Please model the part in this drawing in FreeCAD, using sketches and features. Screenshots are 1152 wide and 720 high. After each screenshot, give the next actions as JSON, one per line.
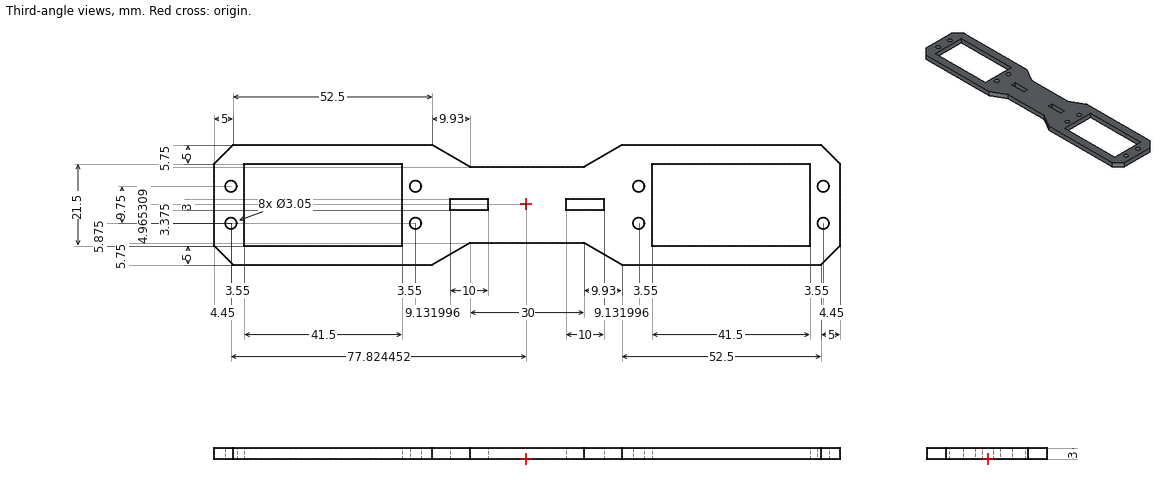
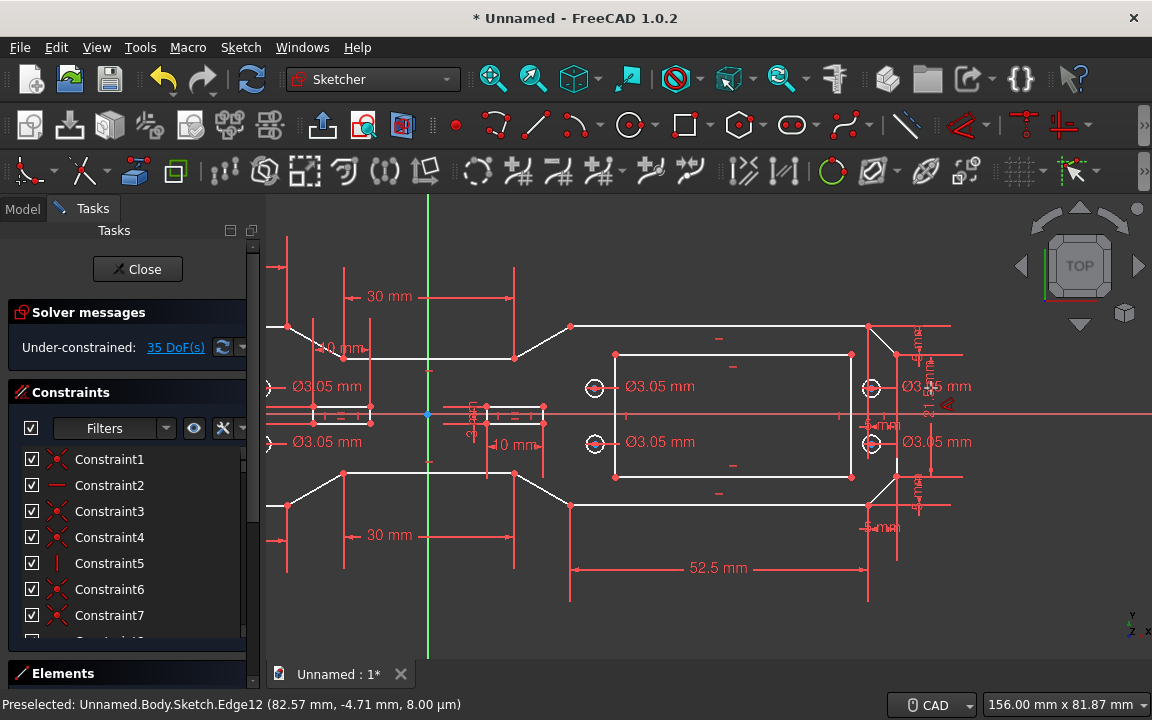
{"action": "left_click", "coordinate": [779, 326]}
{"action": "left_click", "coordinate": [719, 292]}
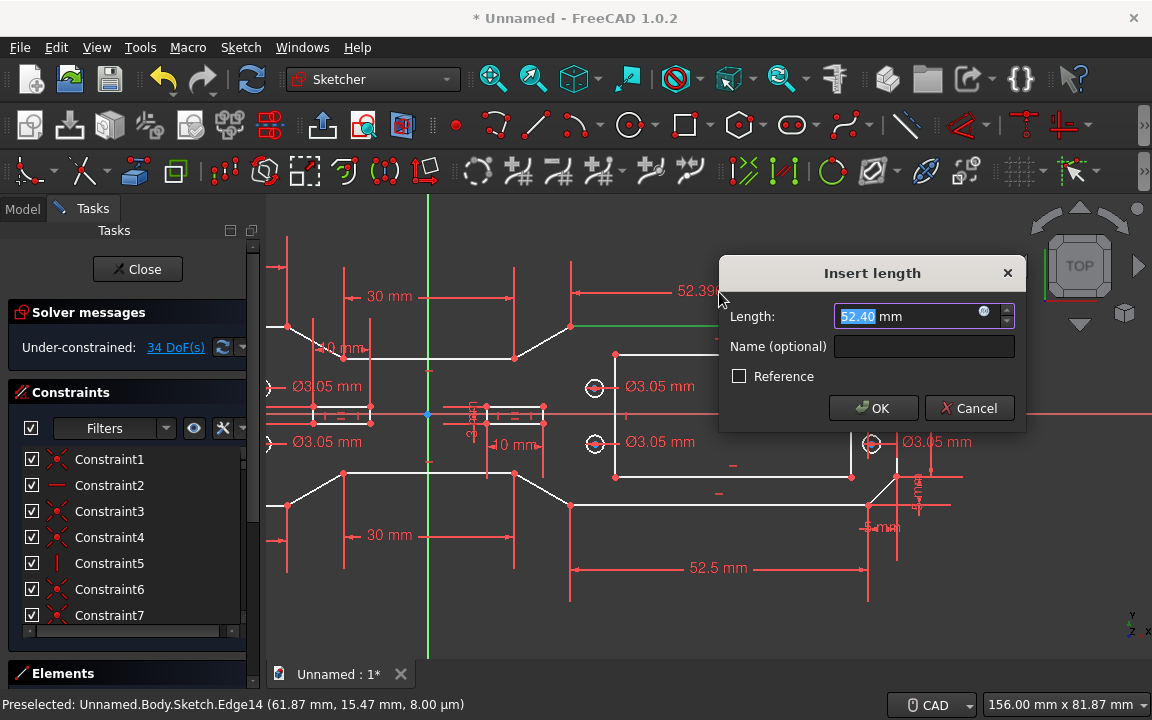
{"action": "type", "text": "52.5"}
{"action": "key", "text": "Return"}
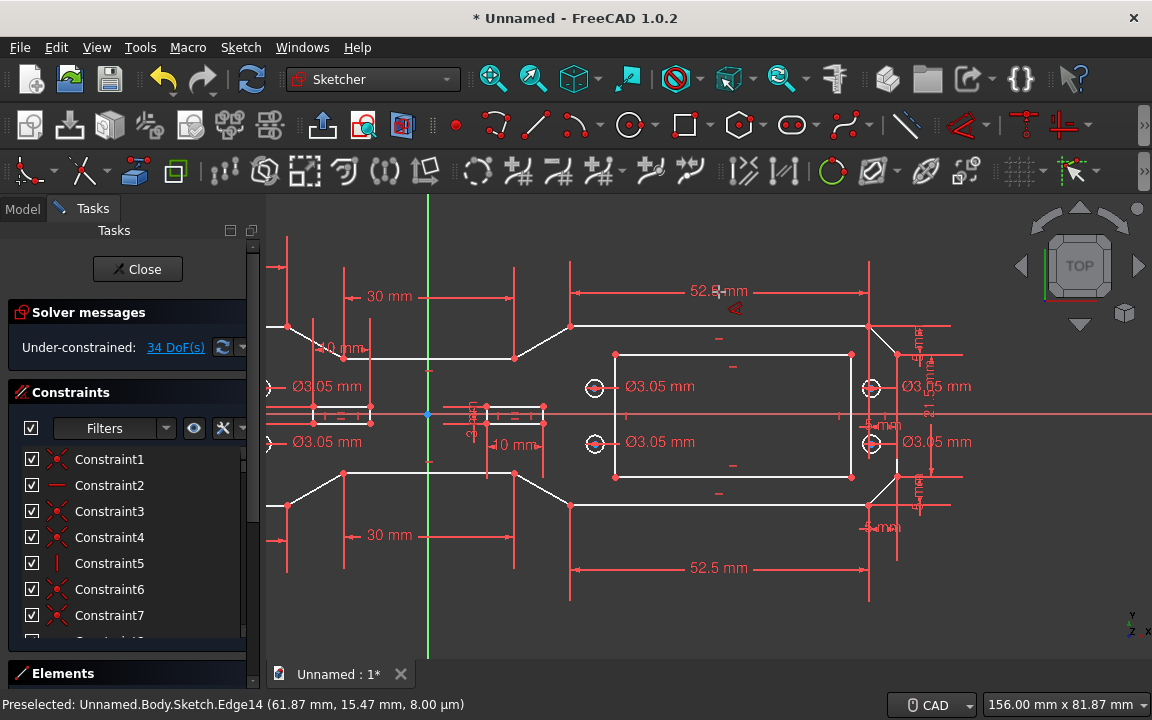
{"action": "left_click", "coordinate": [615, 391]}
{"action": "left_click", "coordinate": [649, 388]}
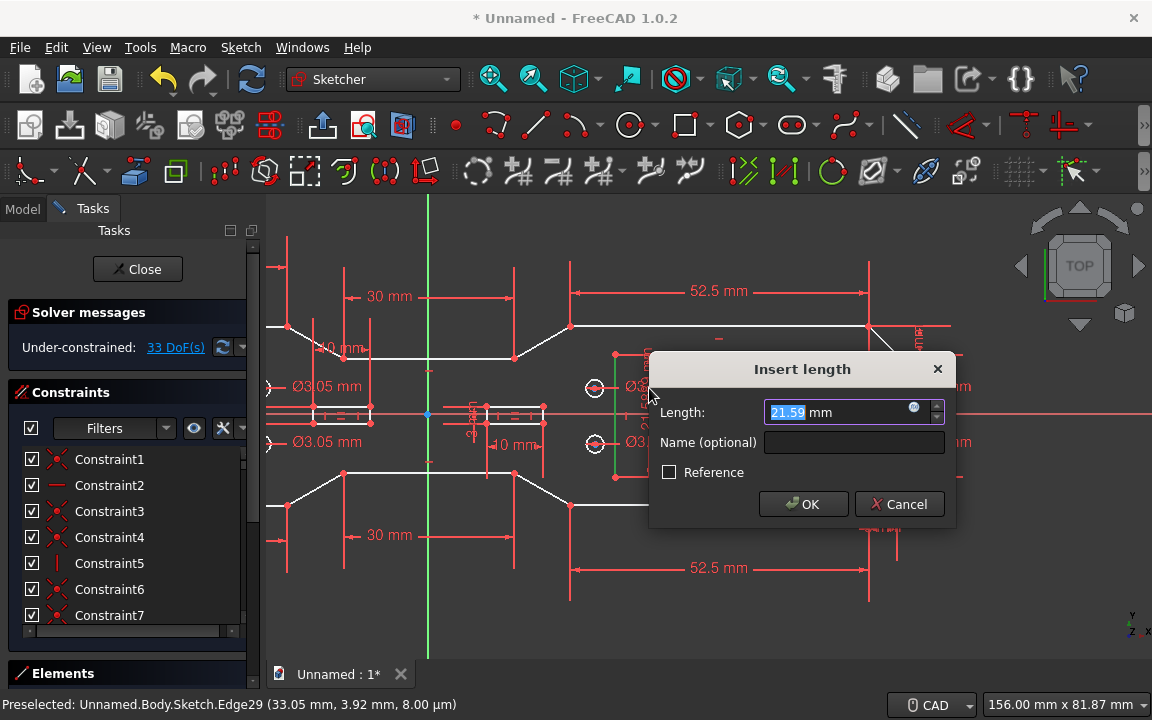
{"action": "type", "text": "21.5"}
{"action": "key", "text": "Return"}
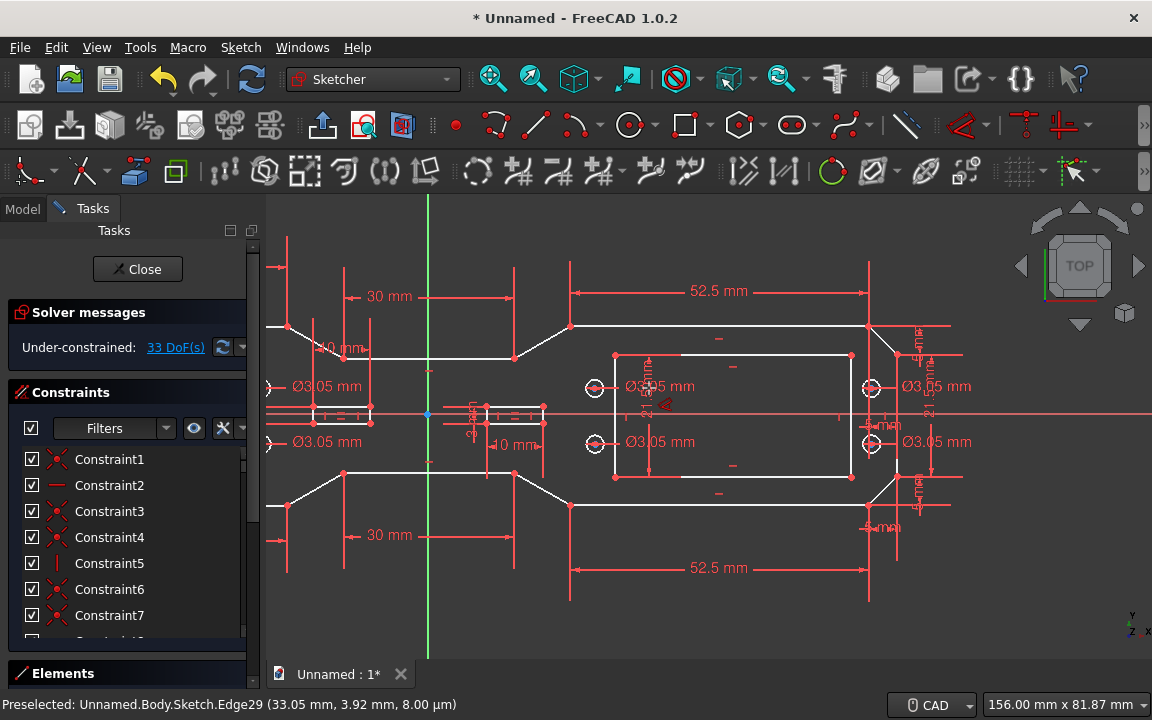
{"action": "left_click", "coordinate": [686, 477]}
{"action": "left_click", "coordinate": [733, 443]}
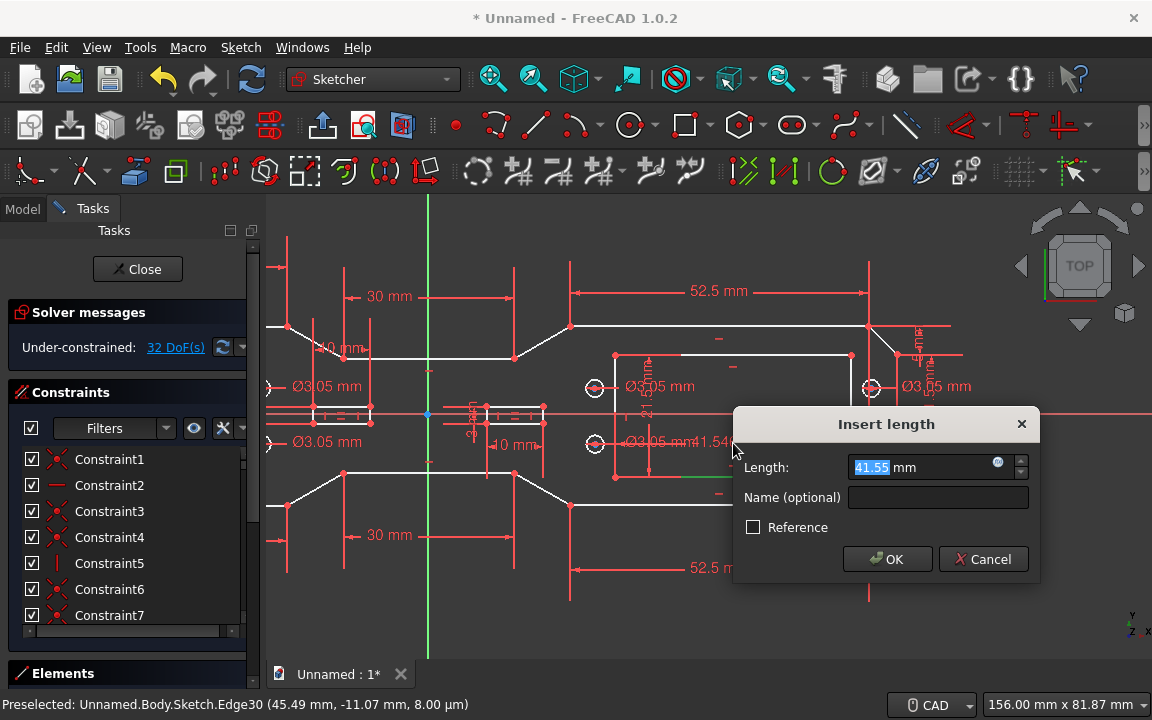
{"action": "type", "text": "41.5"}
{"action": "key", "text": "Return"}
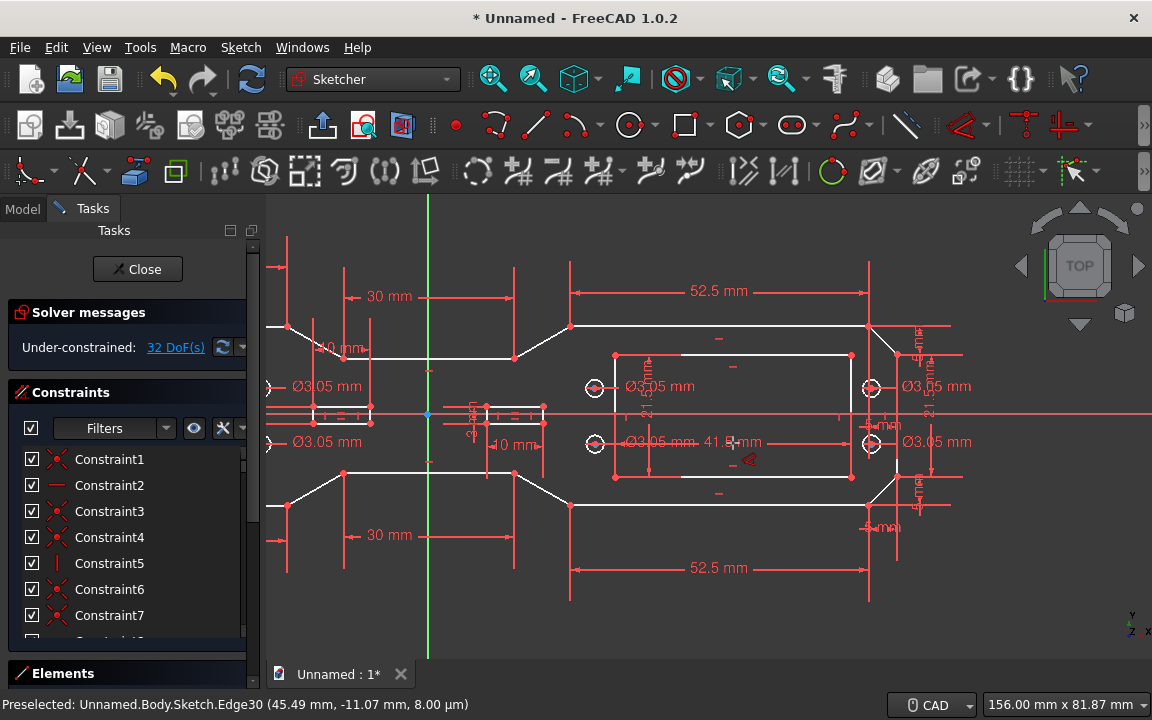
{"action": "left_click", "coordinate": [327, 349]}
{"action": "left_click", "coordinate": [319, 293]}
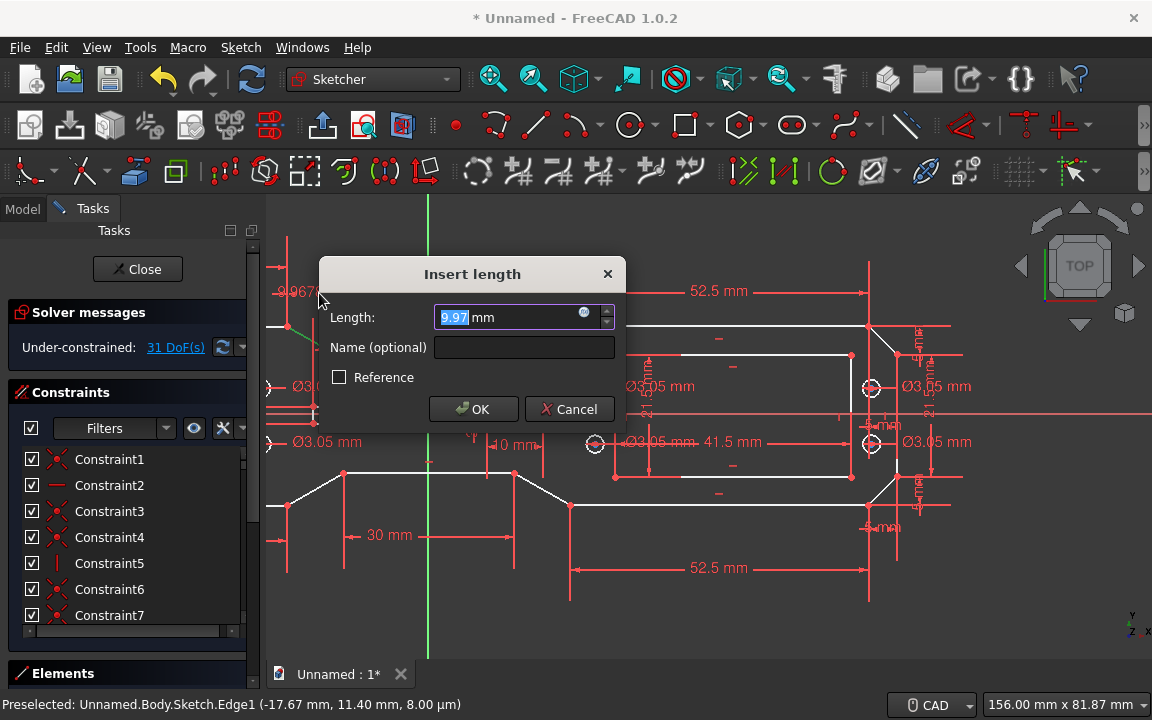
{"action": "type", "text": "9.93"}
{"action": "key", "text": "Return"}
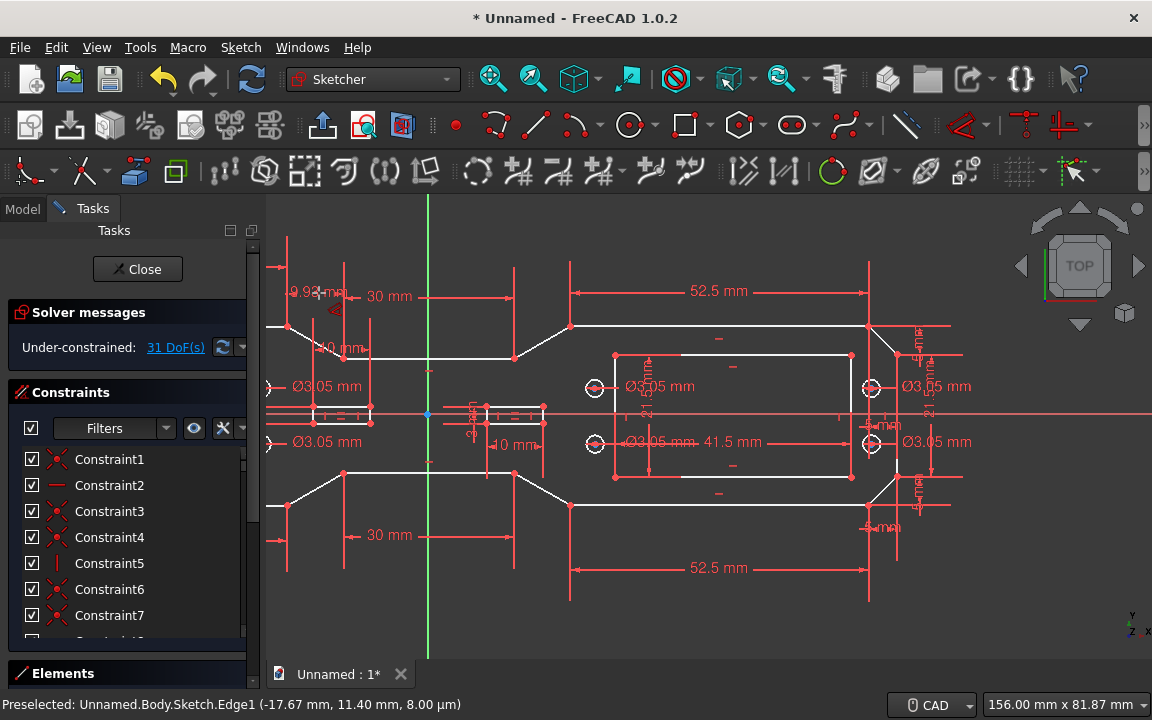
{"action": "left_click", "coordinate": [327, 349]}
{"action": "left_click", "coordinate": [378, 343]}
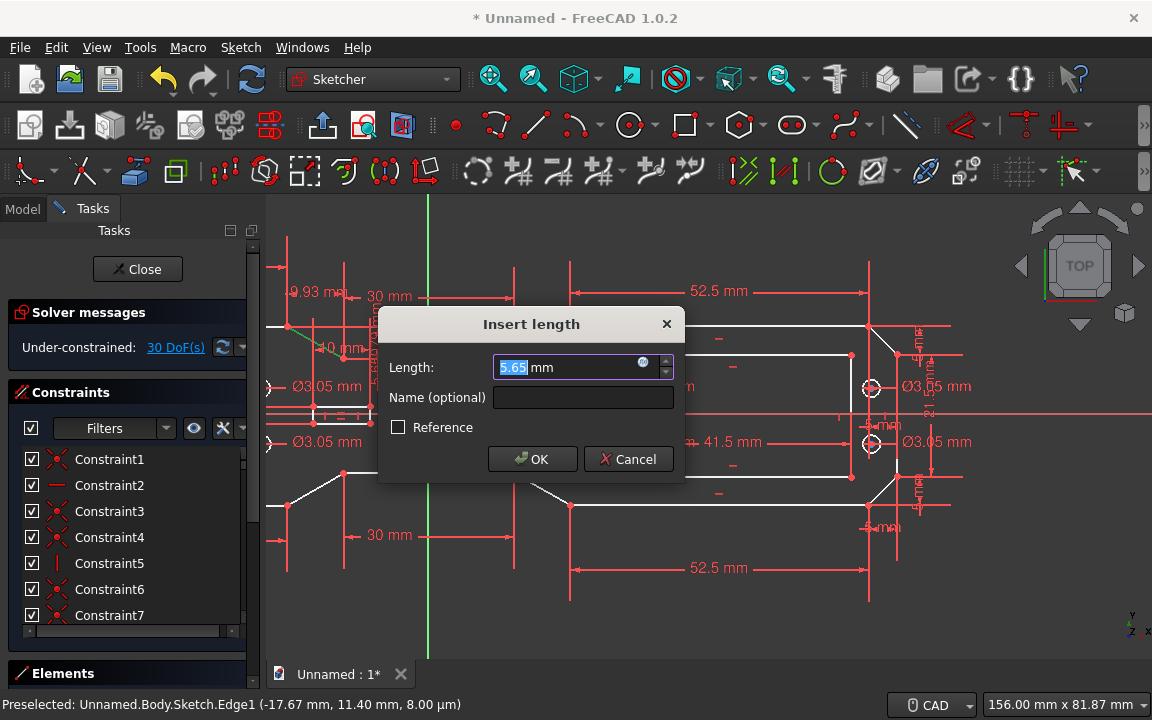
{"action": "type", "text": "5.75"}
{"action": "key", "text": "Return"}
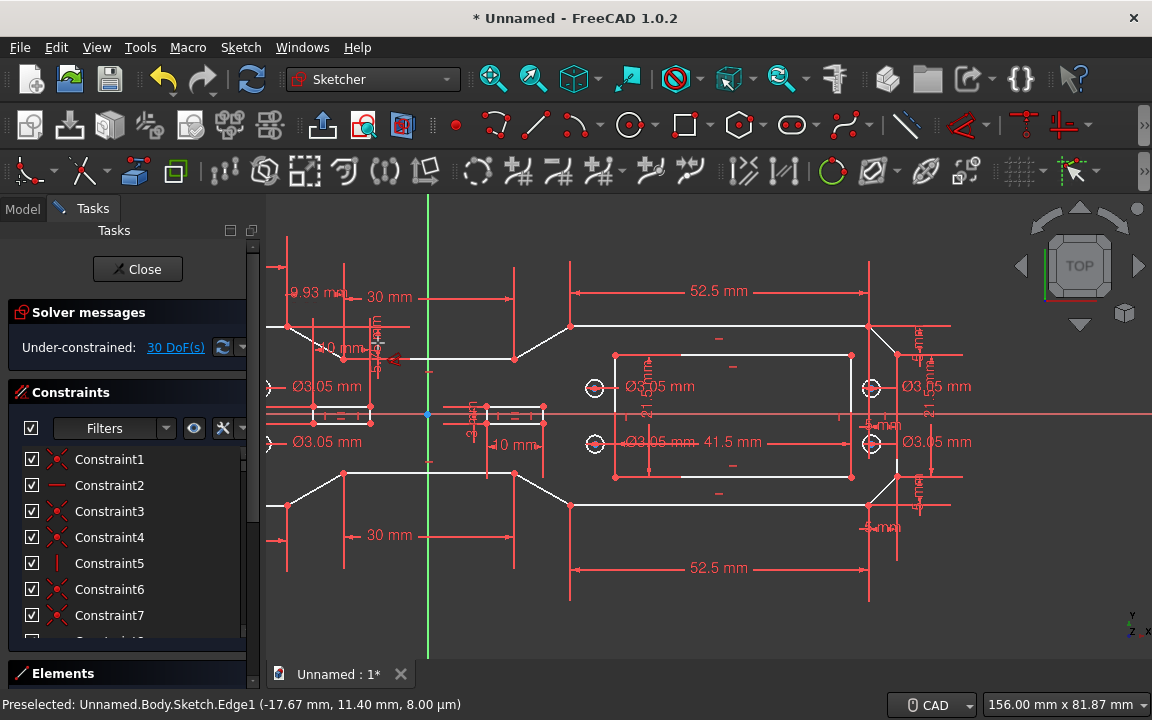
{"action": "left_click", "coordinate": [304, 496]}
{"action": "left_click", "coordinate": [319, 540]}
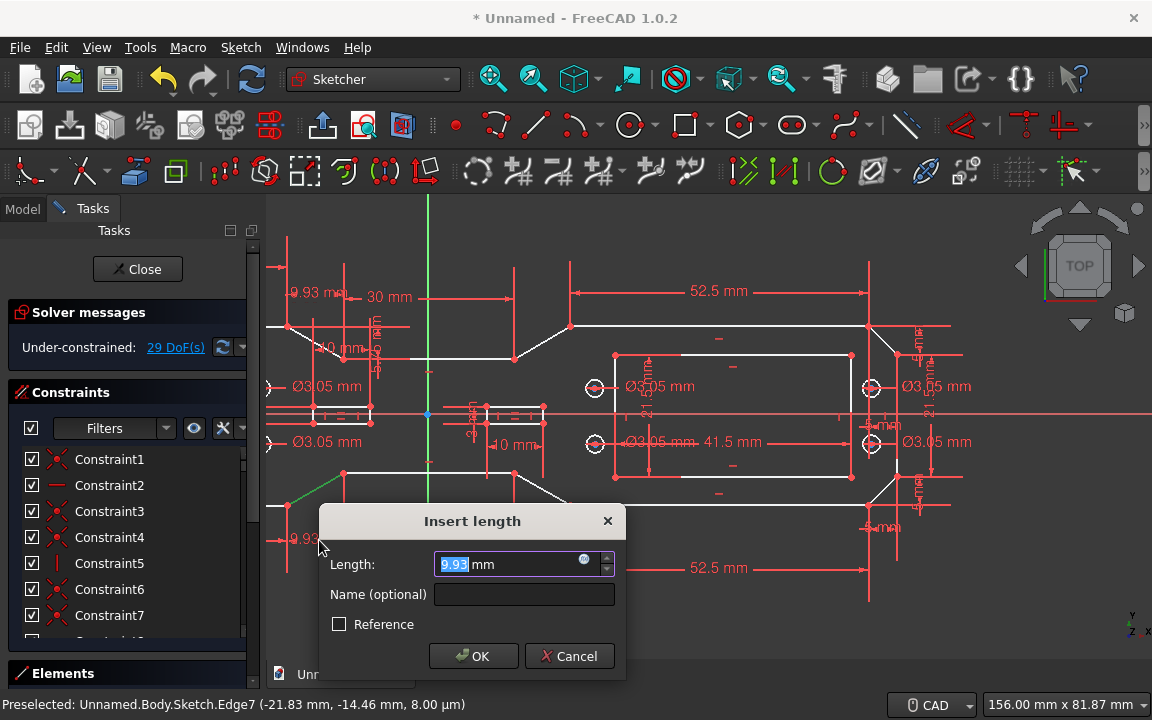
{"action": "type", "text": "9.93"}
{"action": "key", "text": "Return"}